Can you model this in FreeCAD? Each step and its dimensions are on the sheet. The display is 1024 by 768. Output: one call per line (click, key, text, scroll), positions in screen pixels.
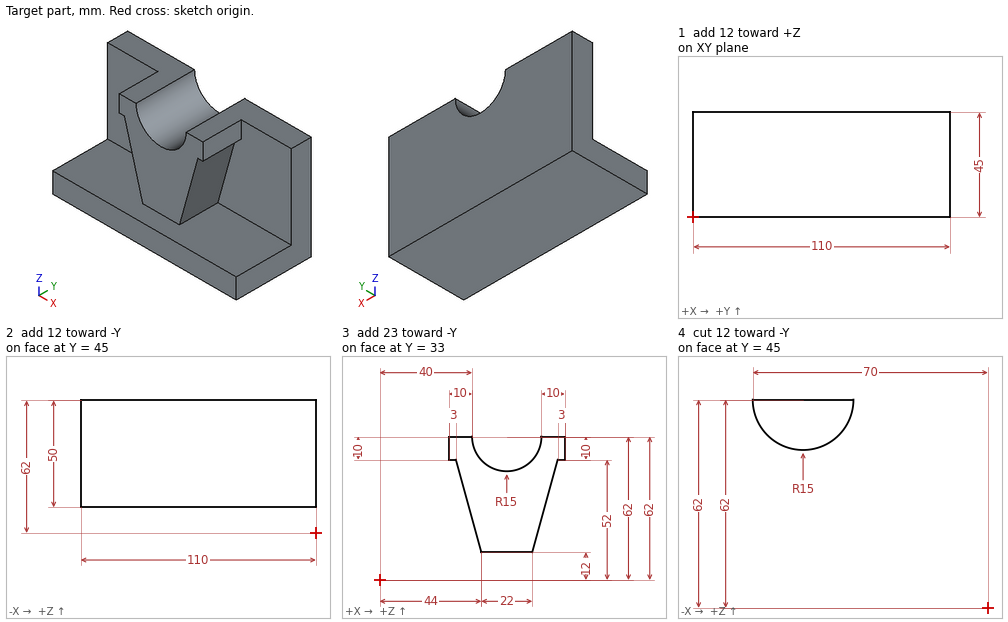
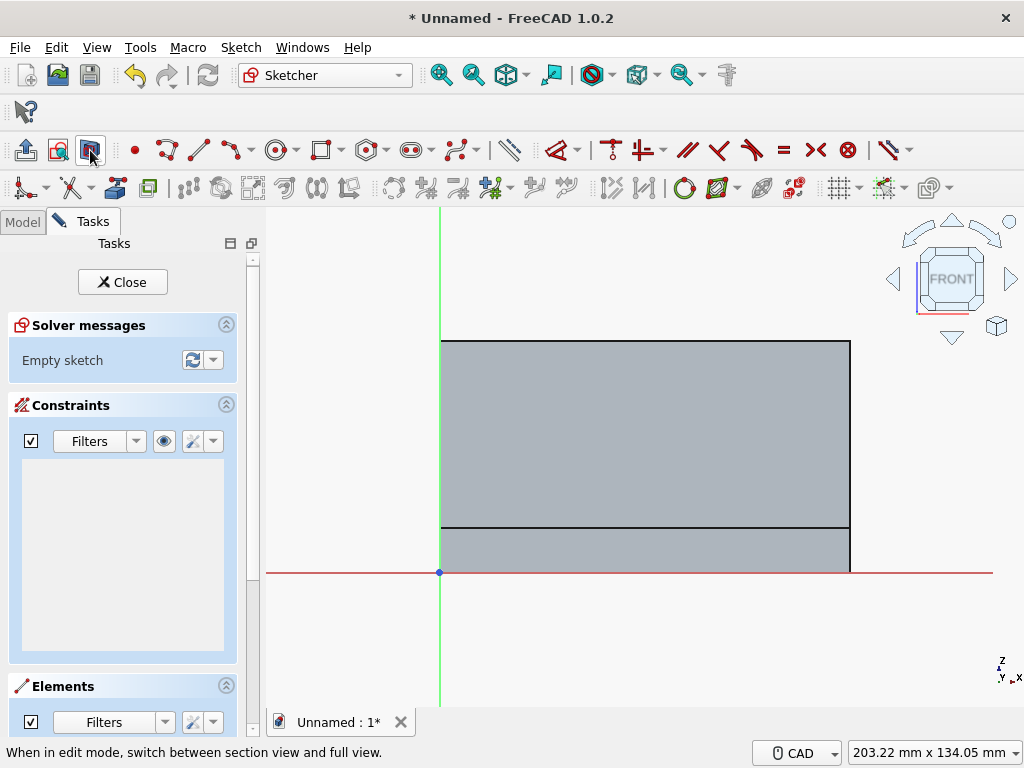
click(168, 150)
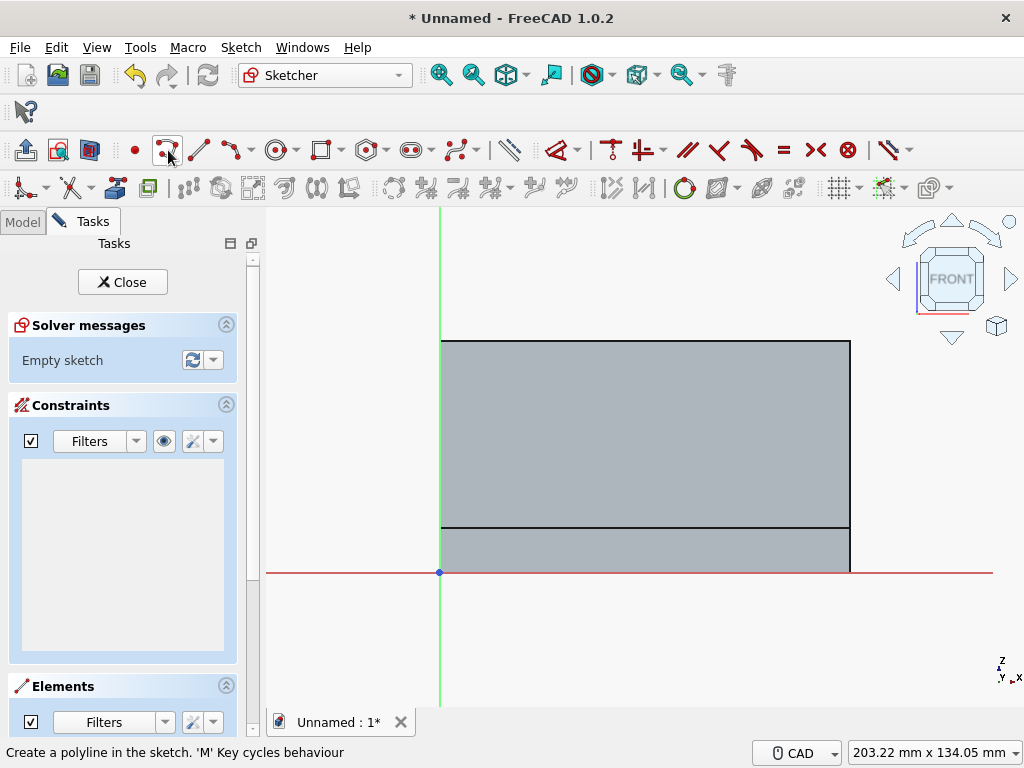
click(589, 341)
click(552, 341)
click(552, 379)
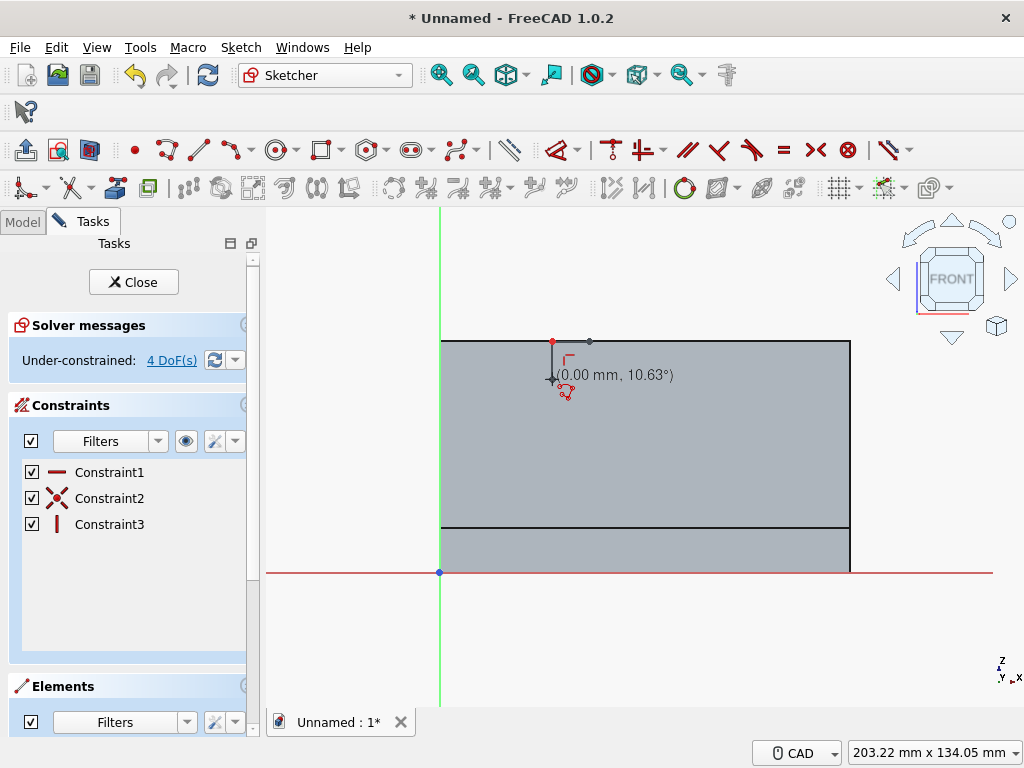
scroll(563, 379, up, 2)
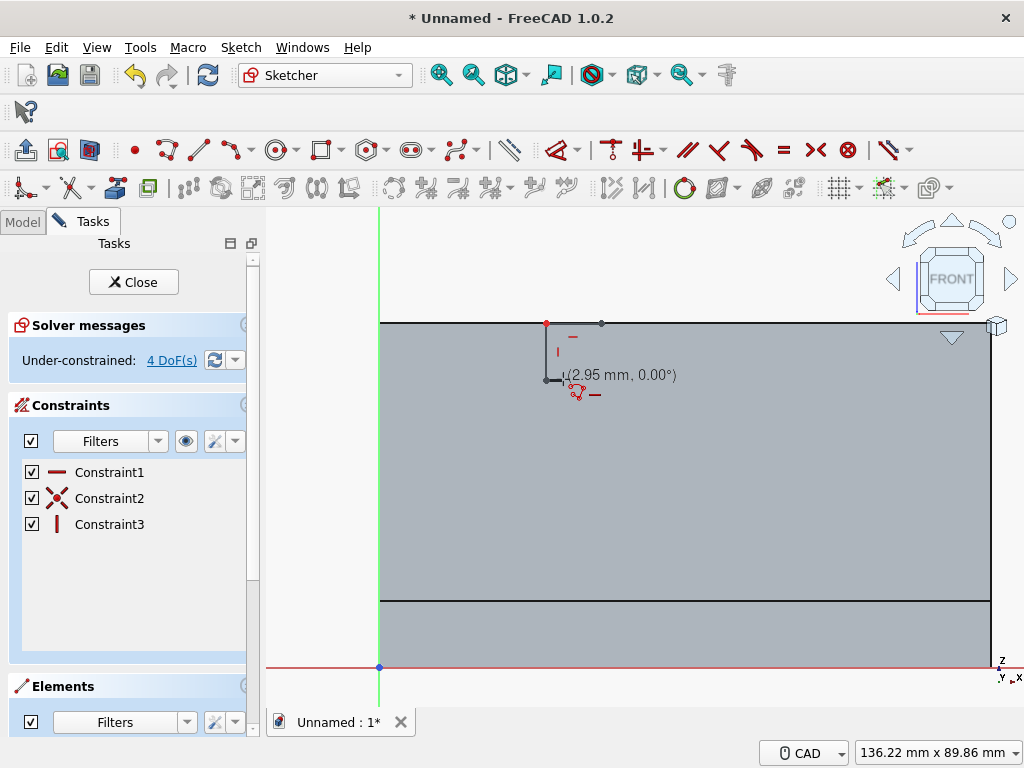
click(563, 379)
click(624, 601)
click(746, 601)
click(808, 378)
click(824, 378)
click(824, 323)
click(769, 323)
right_click(769, 323)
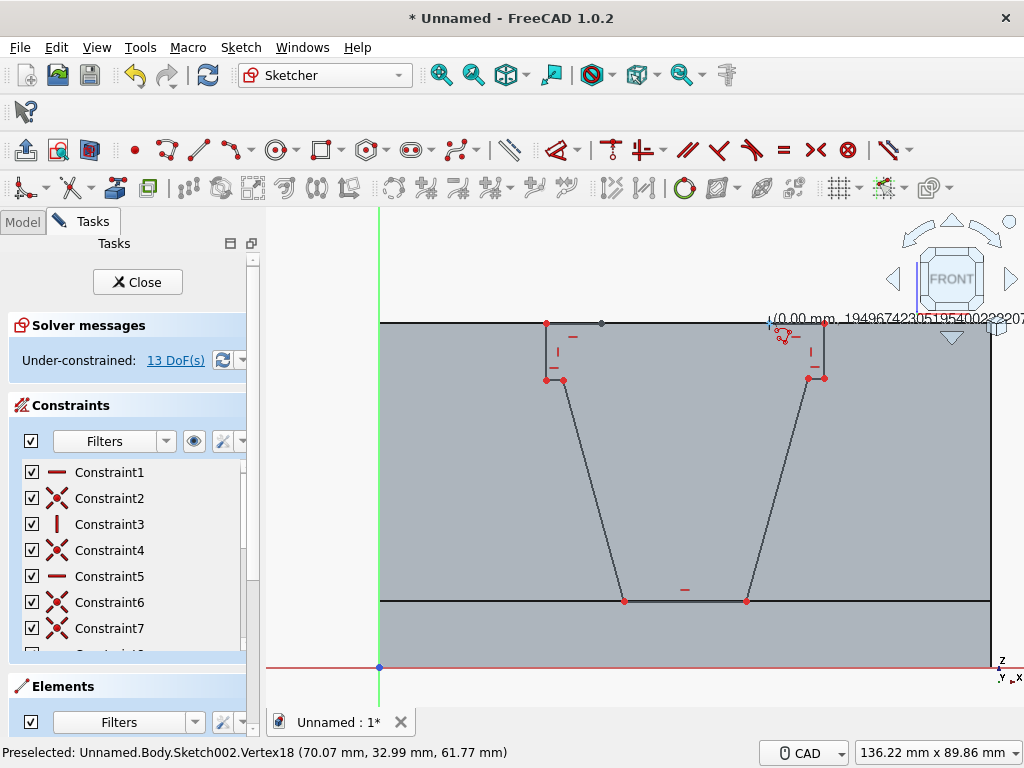
click(232, 150)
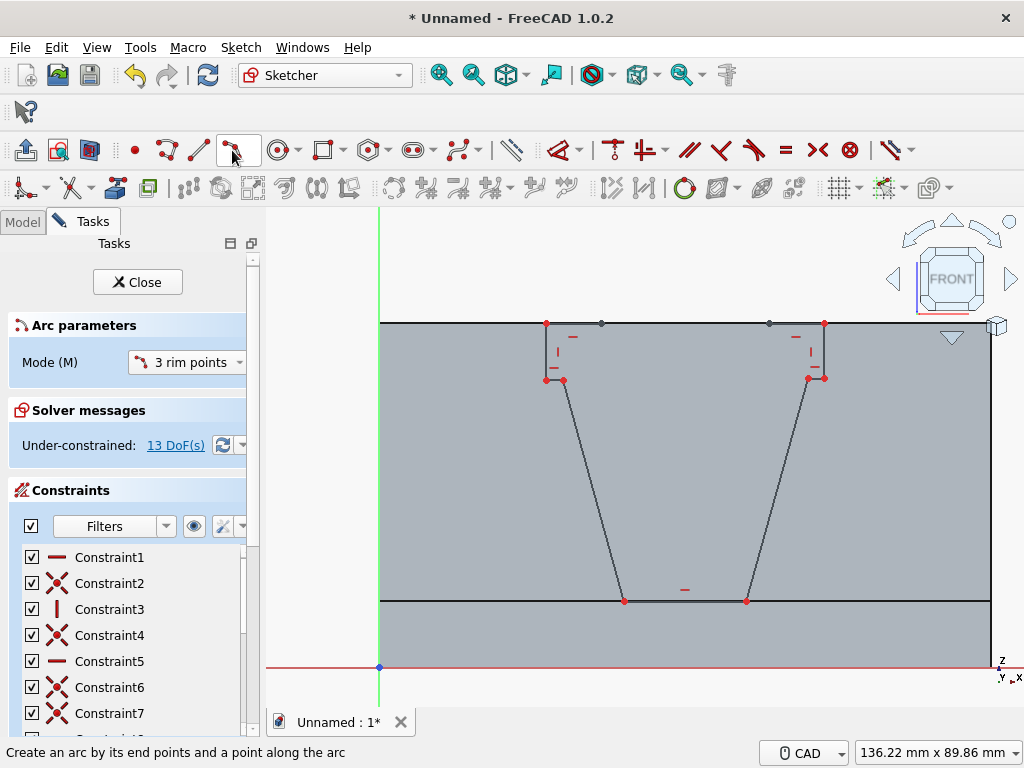
click(769, 324)
click(602, 324)
click(685, 406)
key(Escape)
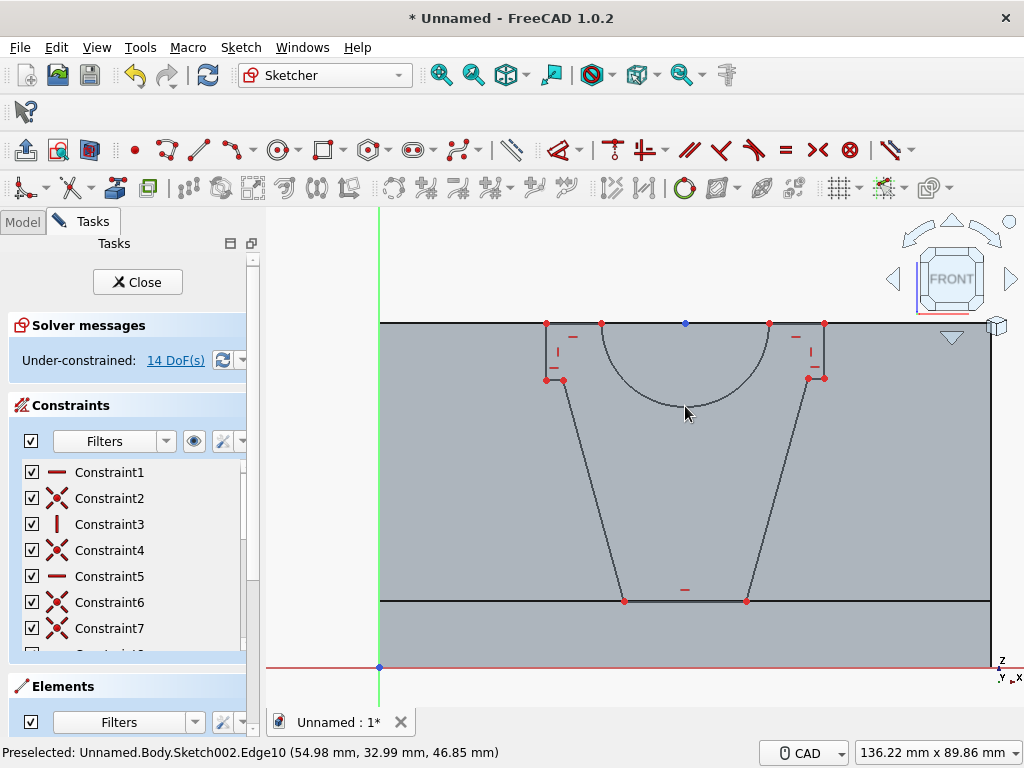
click(558, 150)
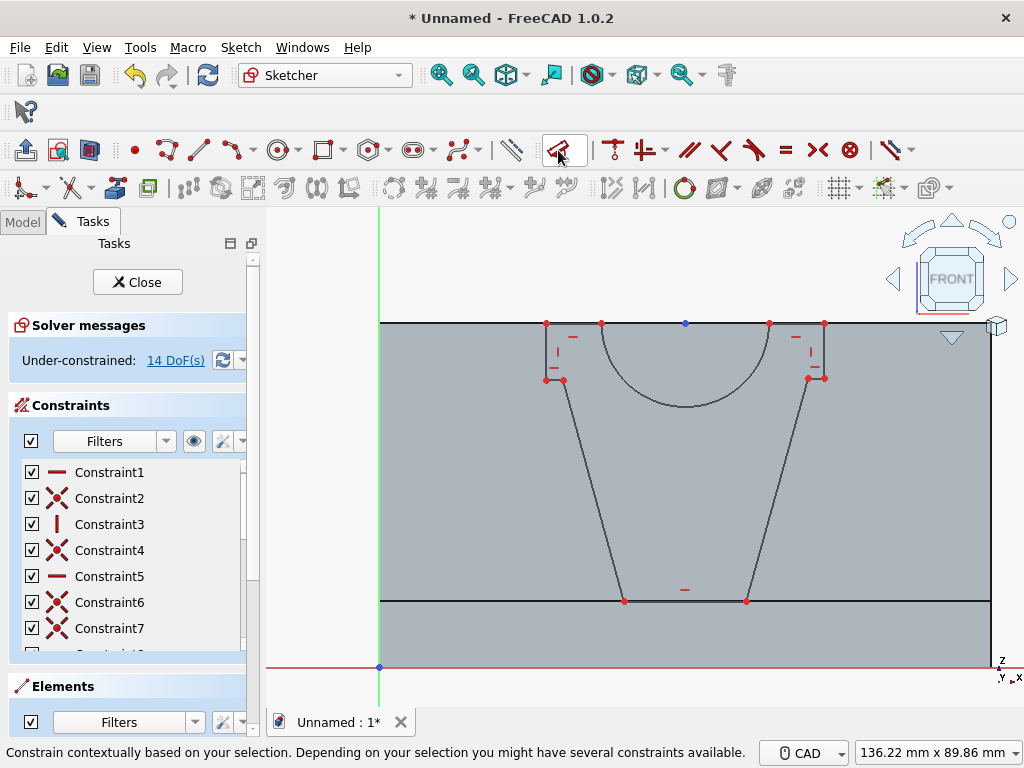
click(636, 391)
click(617, 417)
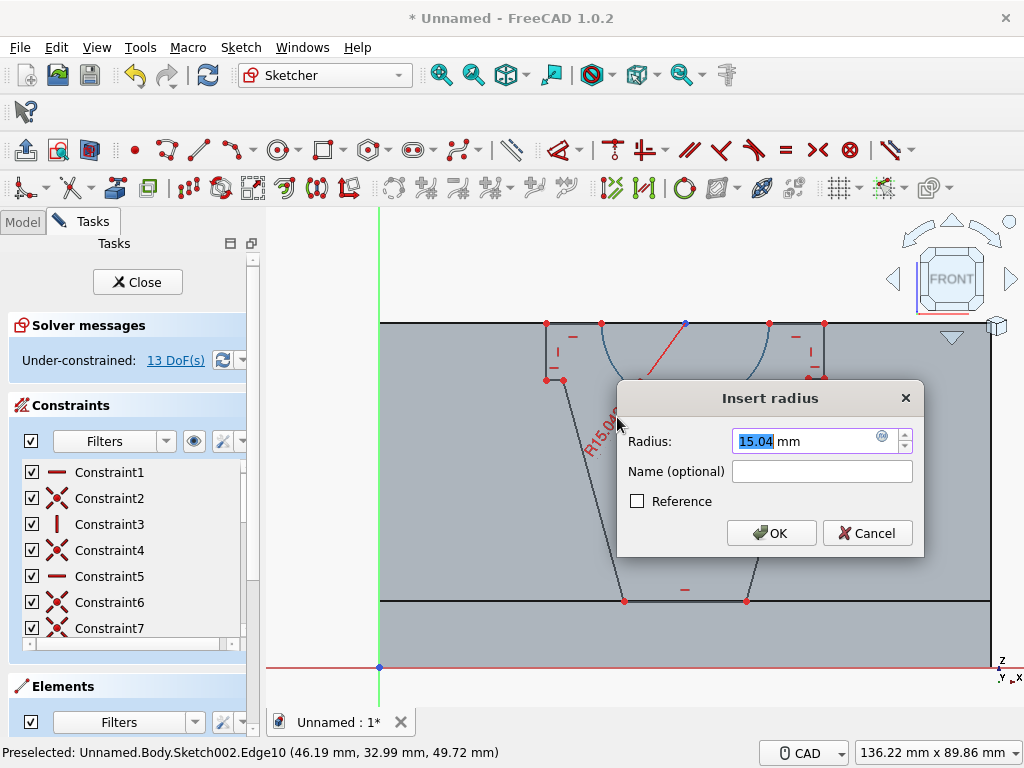
text(15)
key(Return)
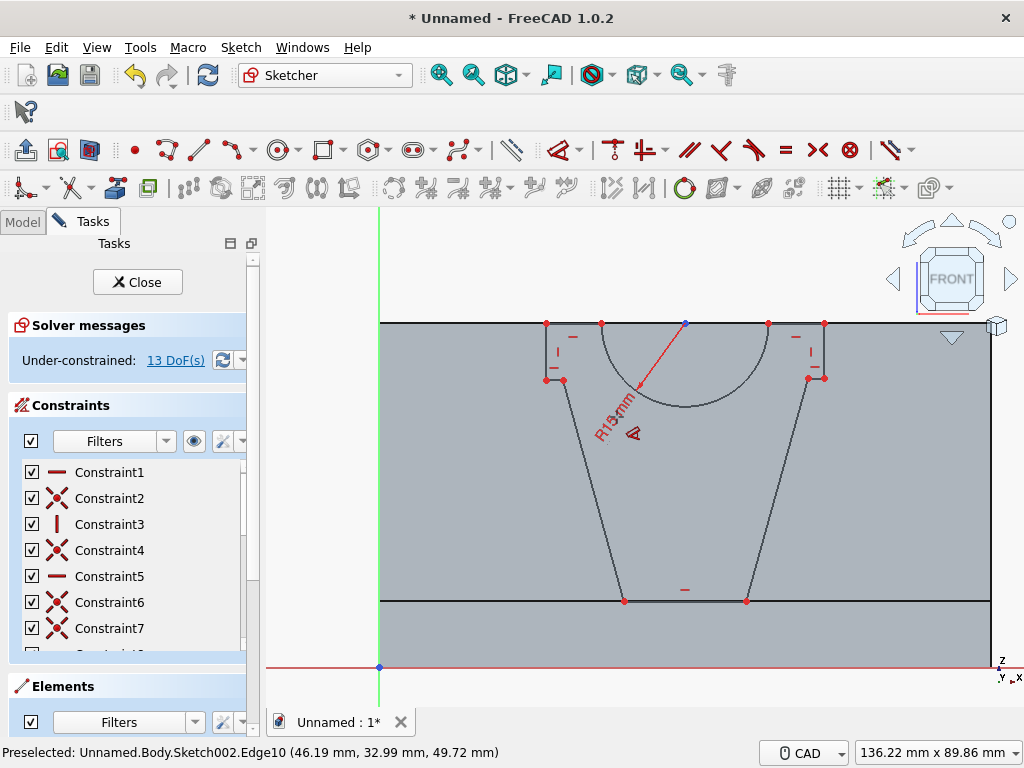
scroll(555, 380, up, 5)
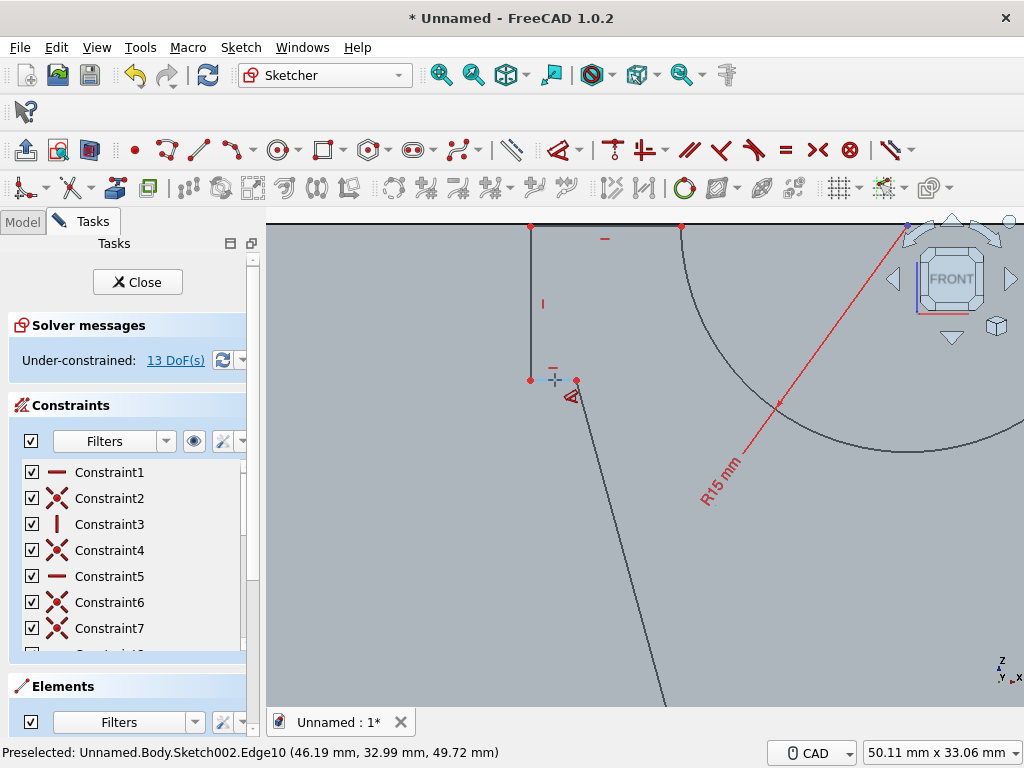
click(554, 380)
click(554, 346)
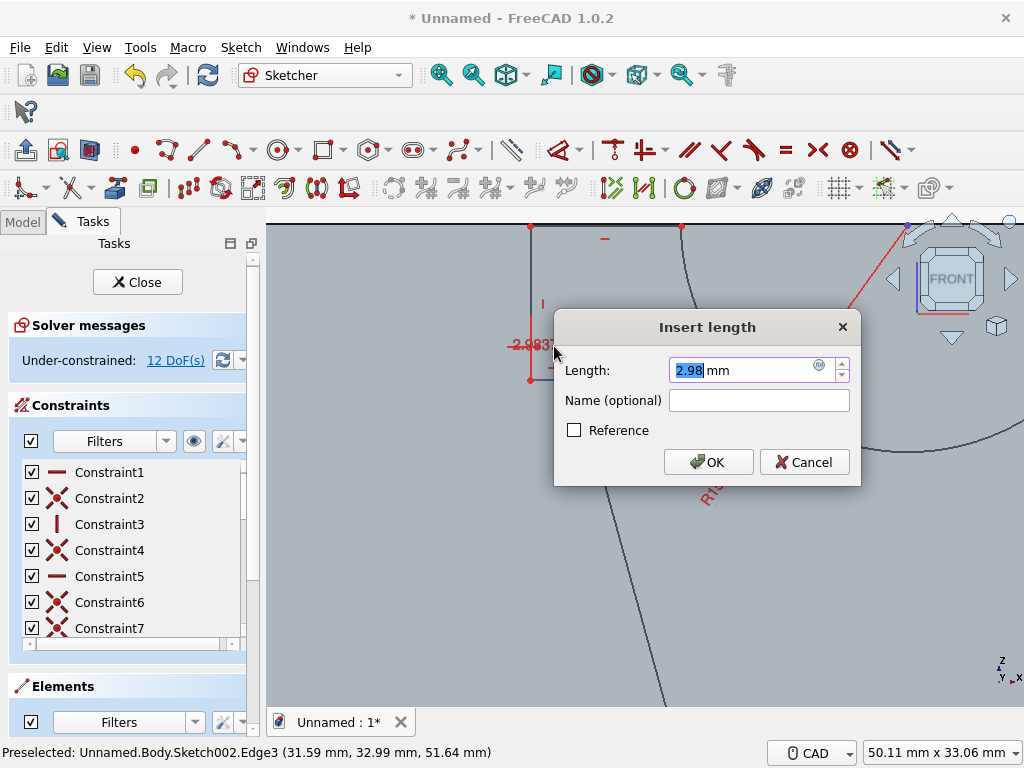
text(3)
key(Return)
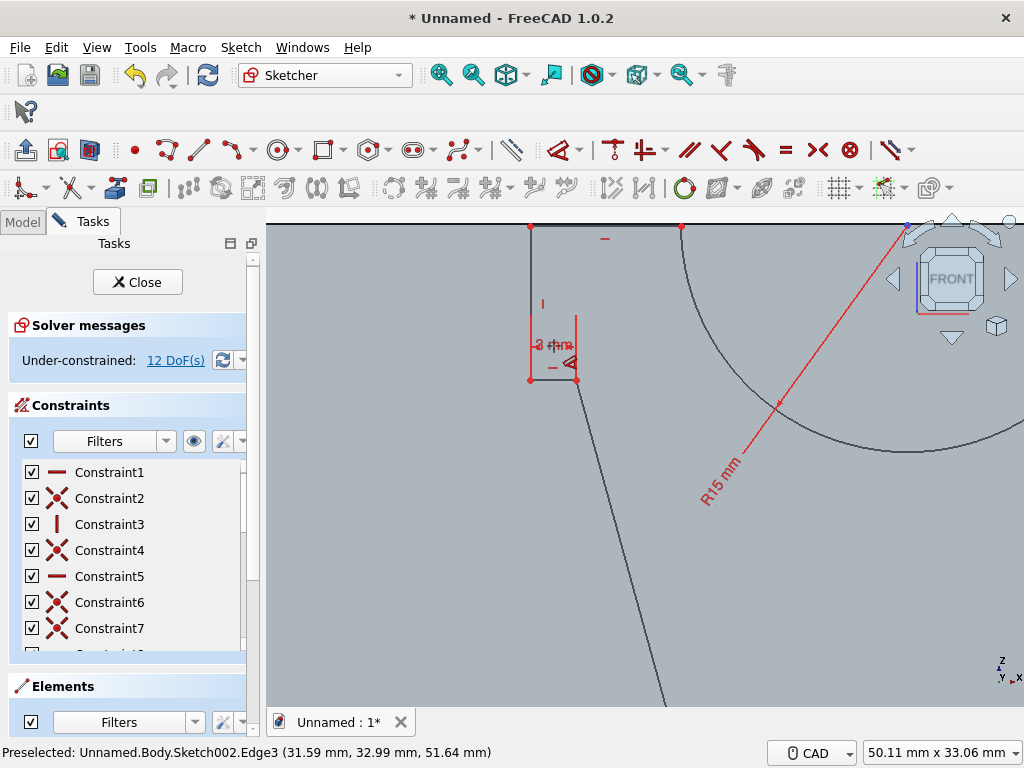
scroll(531, 355, down, 6)